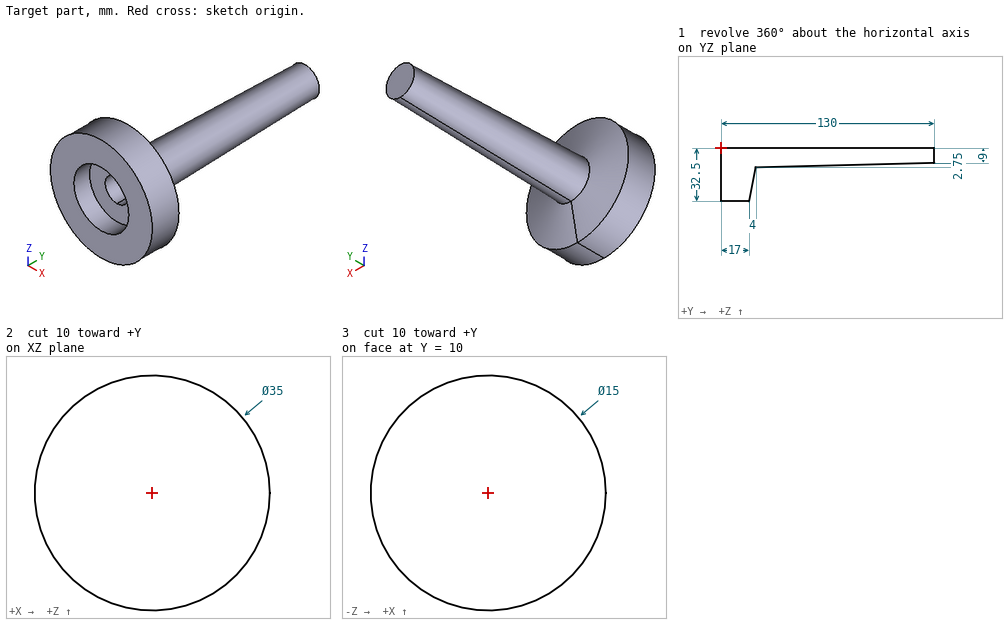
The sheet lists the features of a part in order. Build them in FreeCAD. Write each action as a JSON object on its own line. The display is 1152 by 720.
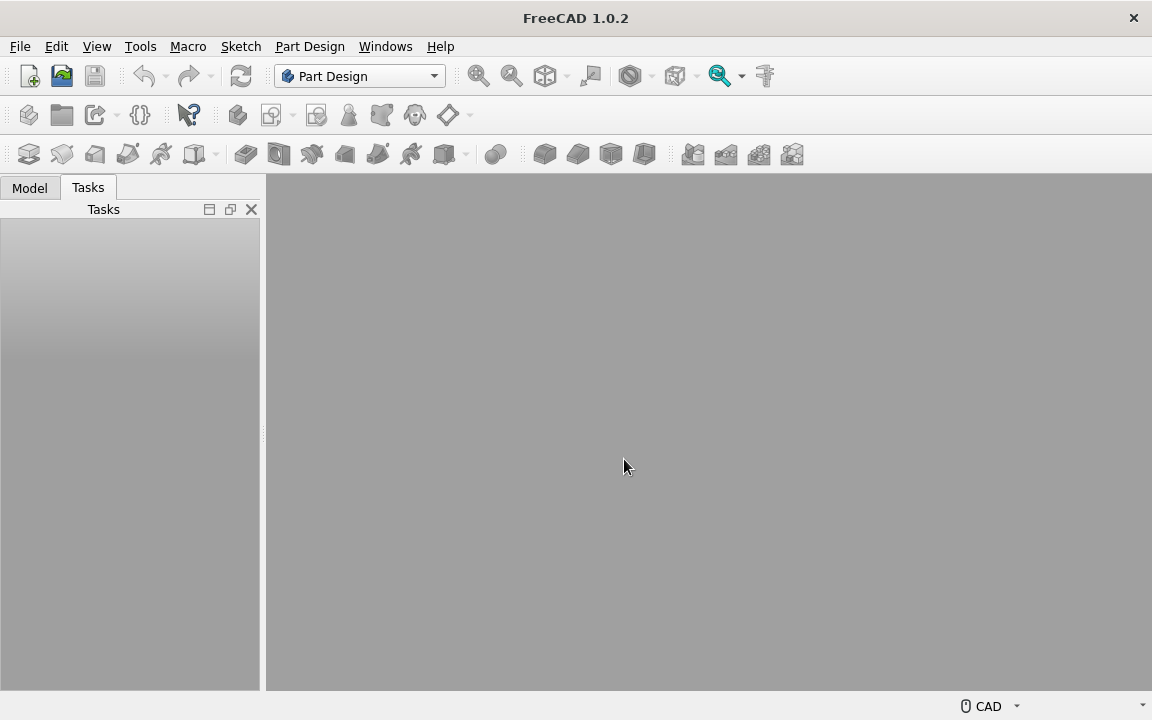
{"action": "left_click", "coordinate": [29, 76]}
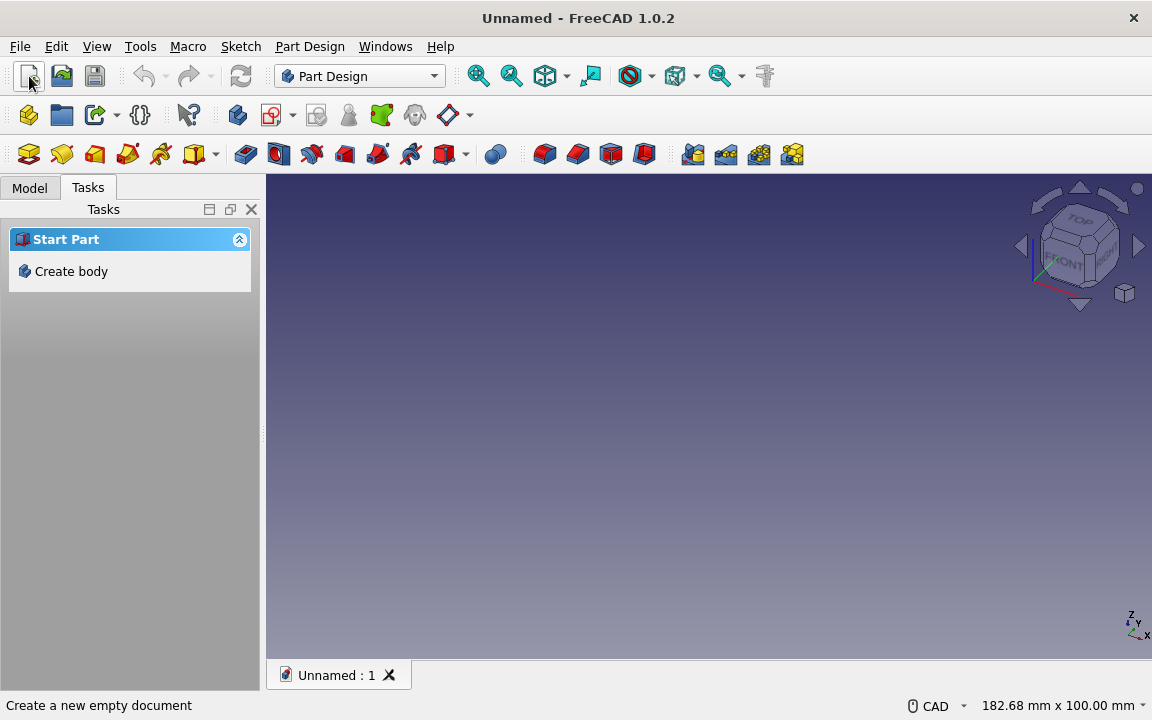
{"action": "left_click", "coordinate": [270, 116]}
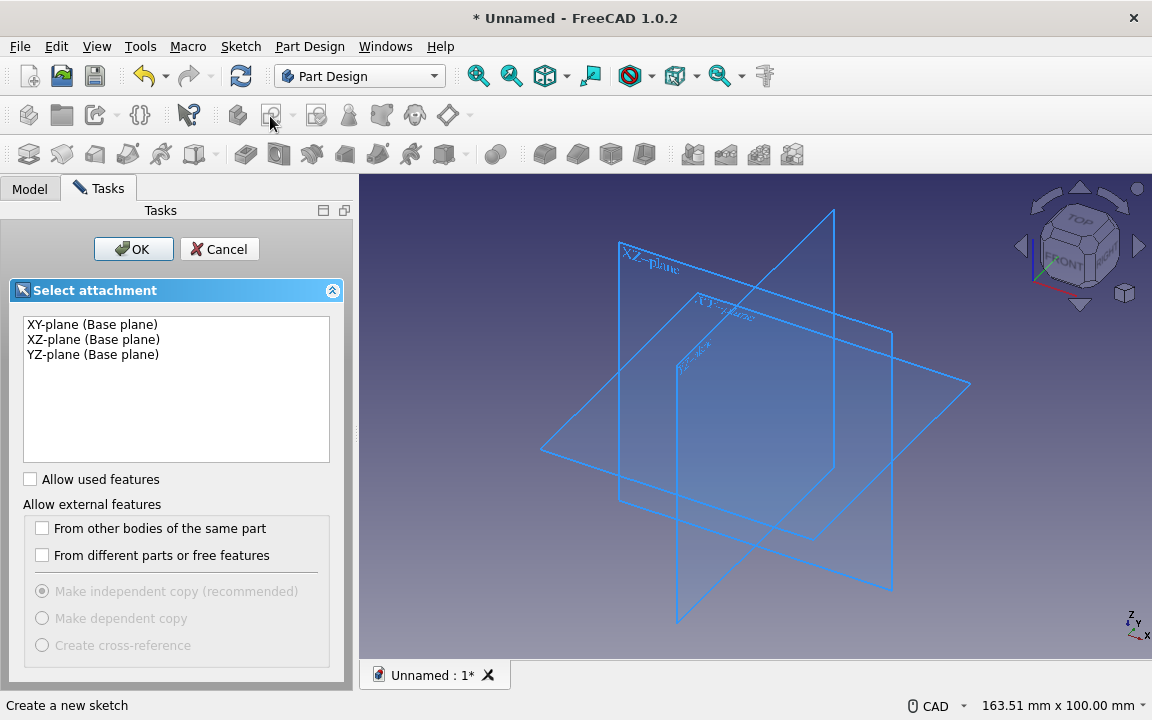
{"action": "left_click", "coordinate": [84, 354]}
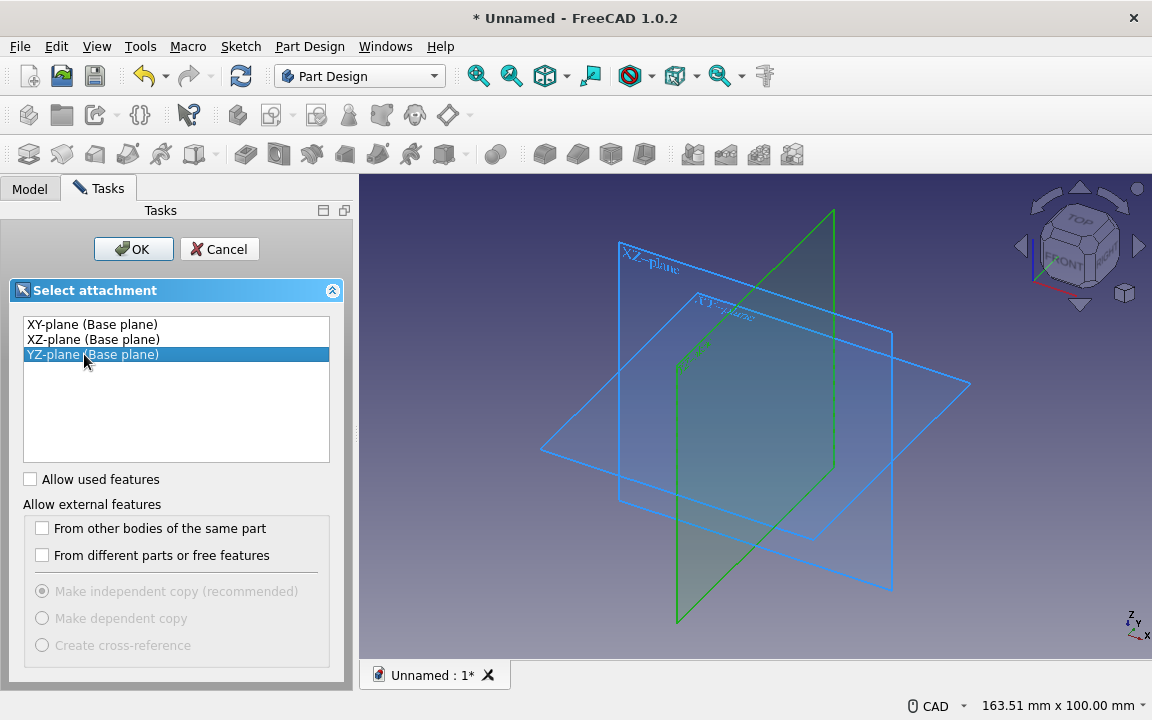
{"action": "left_click", "coordinate": [134, 249]}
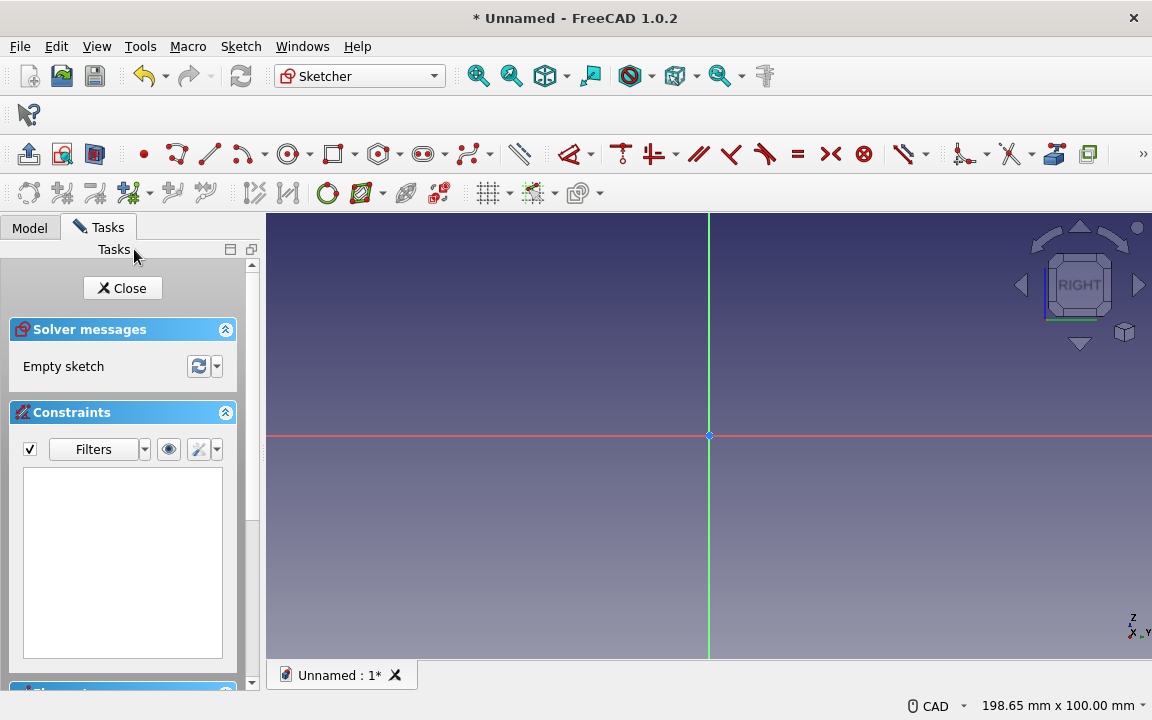
{"action": "scroll", "coordinate": [294, 289], "scroll_direction": "down", "scroll_amount": 2}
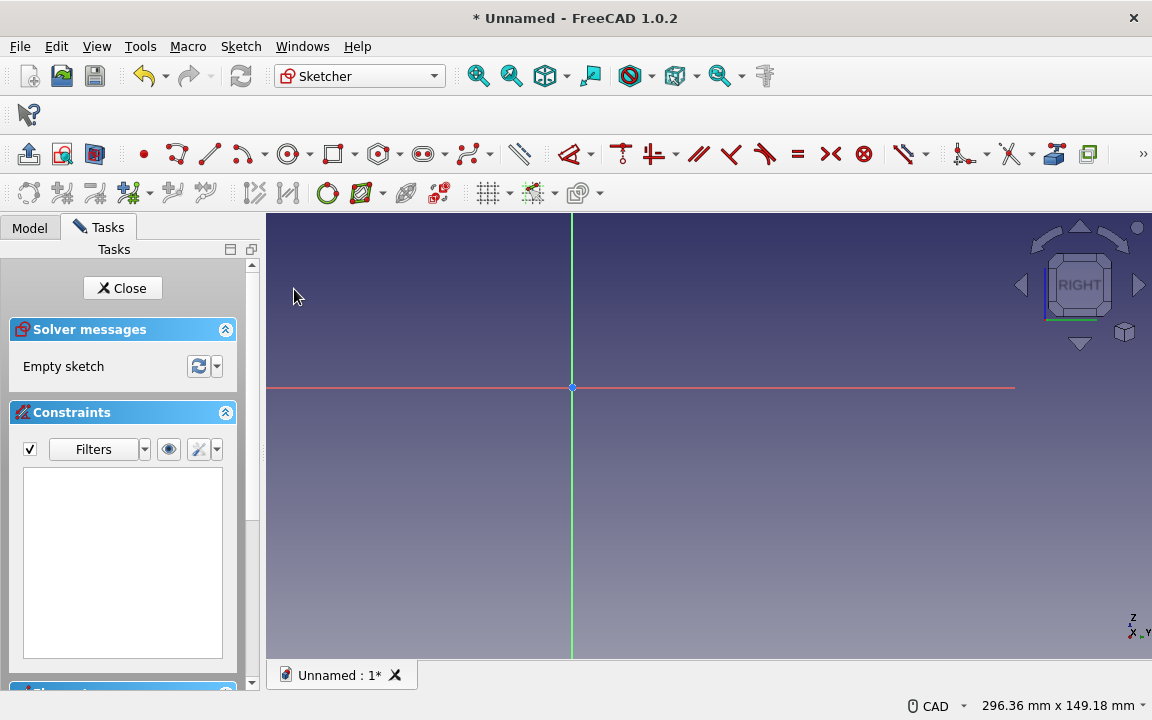
{"action": "left_click", "coordinate": [177, 154]}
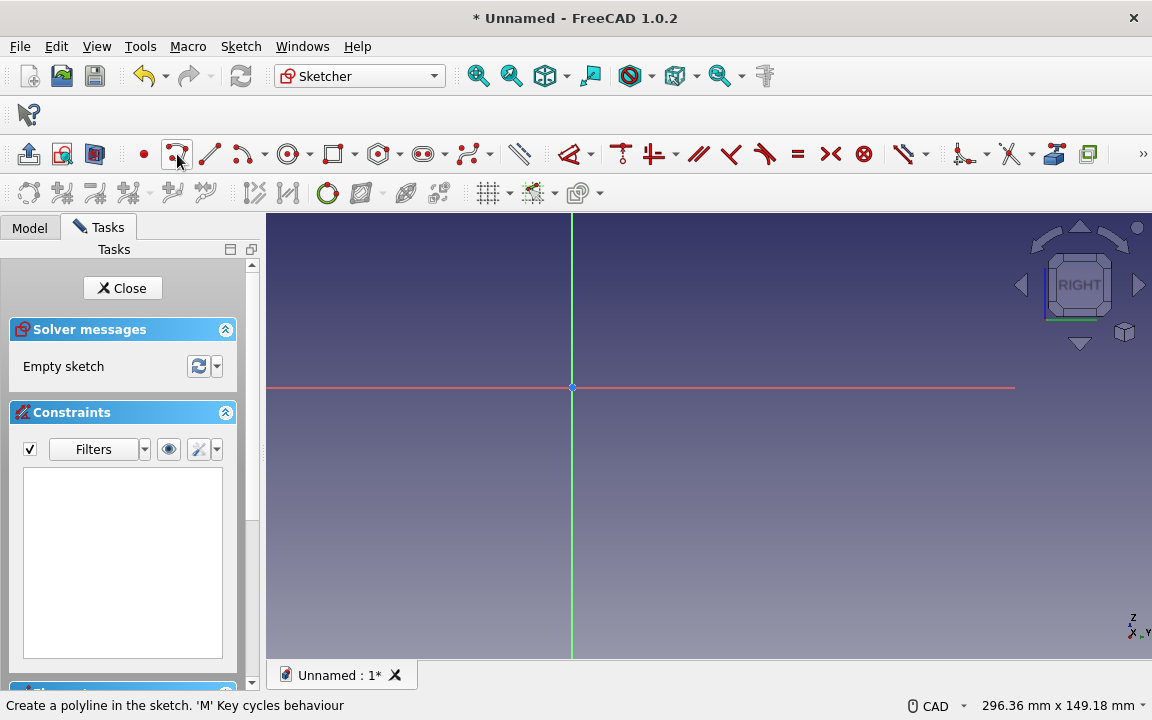
{"action": "left_click", "coordinate": [572, 388]}
{"action": "left_click", "coordinate": [581, 485]}
{"action": "left_click", "coordinate": [623, 485]}
{"action": "left_click", "coordinate": [635, 423]}
{"action": "left_click", "coordinate": [961, 407]}
{"action": "left_click", "coordinate": [961, 397]}
{"action": "left_click", "coordinate": [572, 388]}
{"action": "key", "text": "Escape"}
{"action": "key", "text": "Escape"}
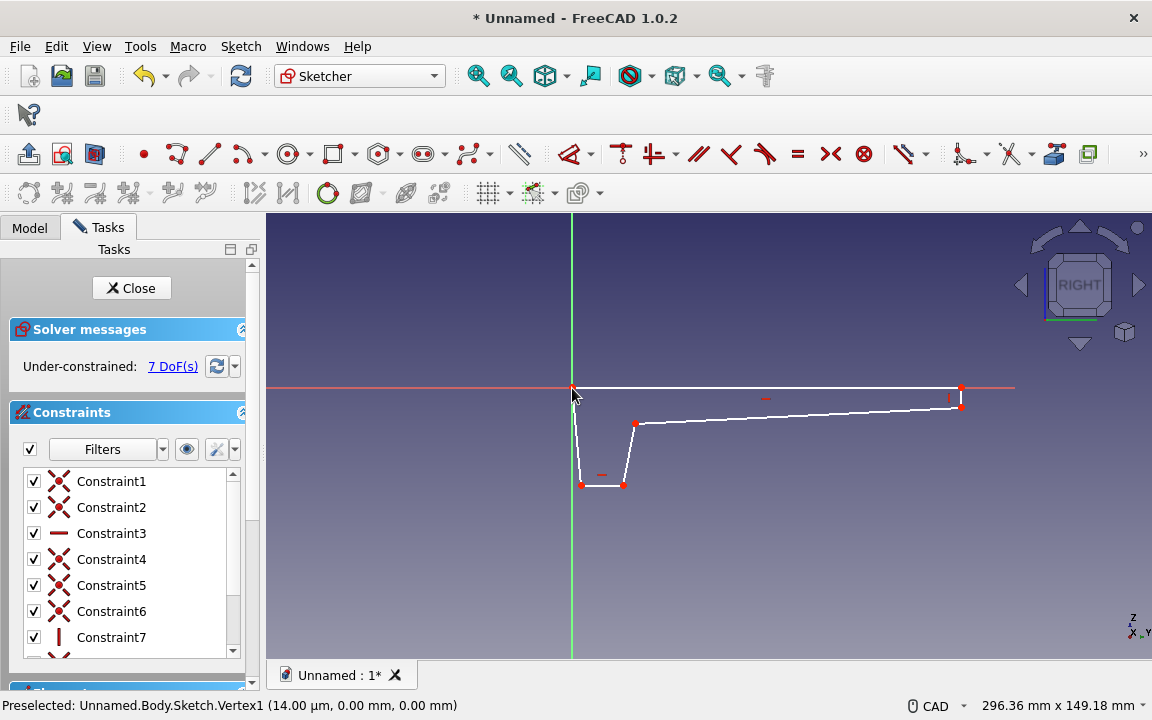
{"action": "left_click", "coordinate": [575, 417]}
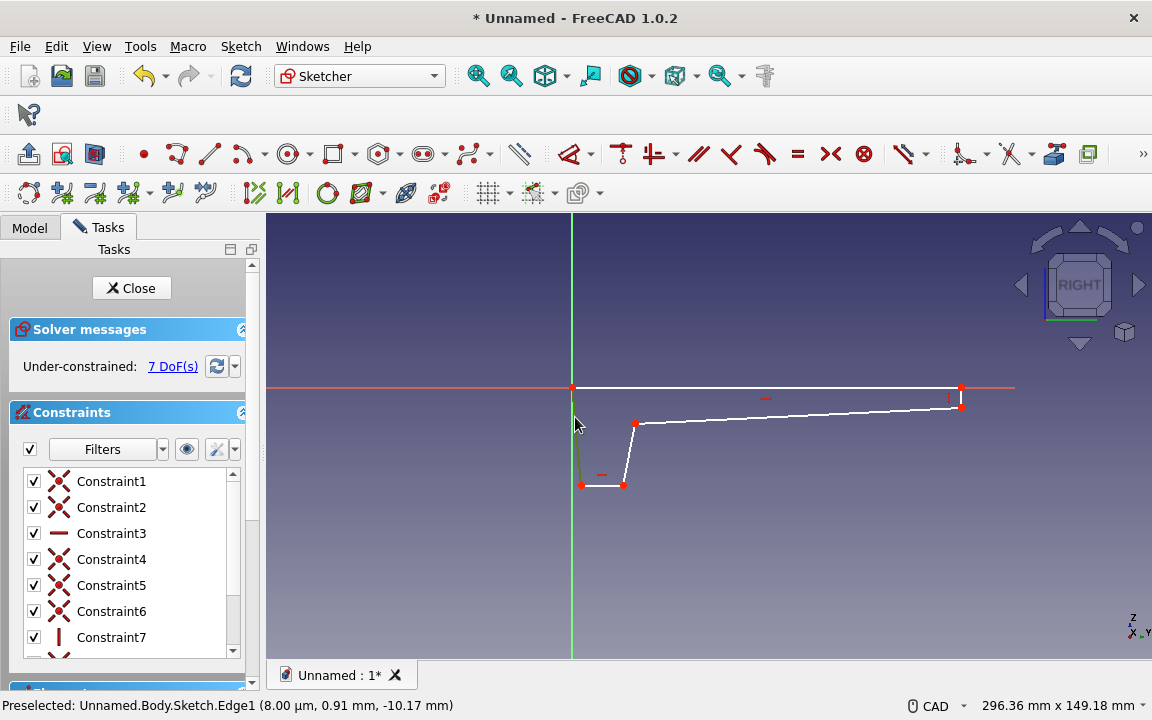
{"action": "key", "text": "v"}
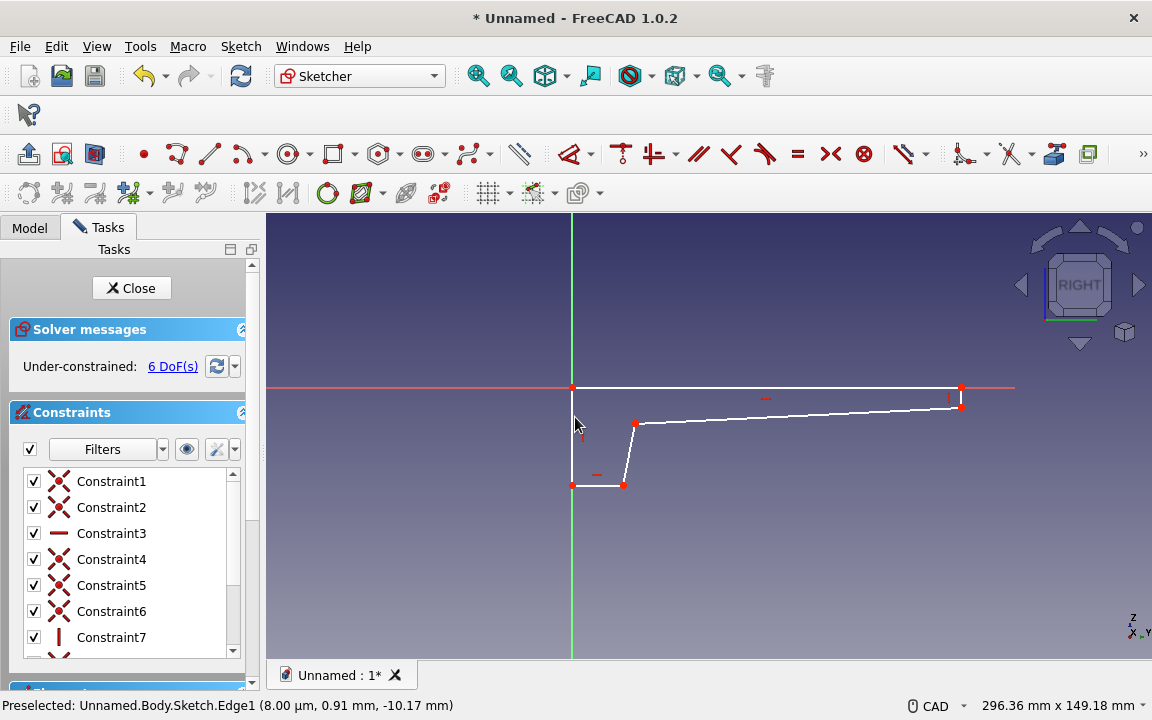
{"action": "left_click", "coordinate": [568, 154]}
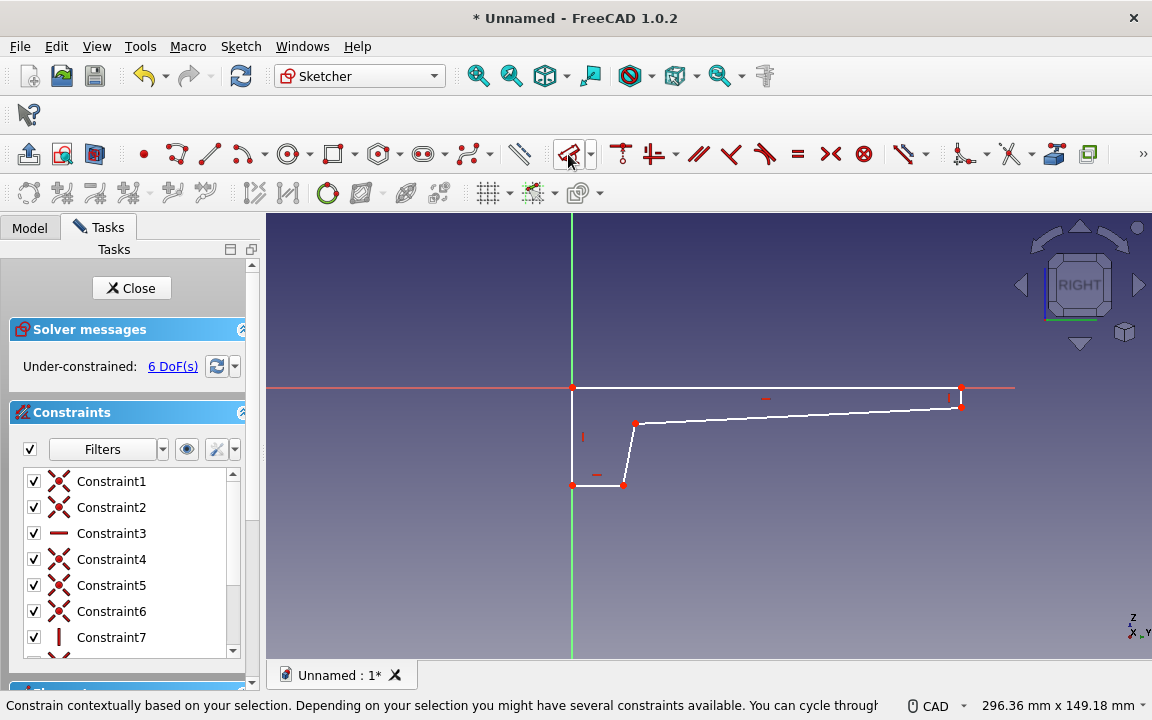
{"action": "scroll", "coordinate": [961, 398], "scroll_direction": "up", "scroll_amount": 2}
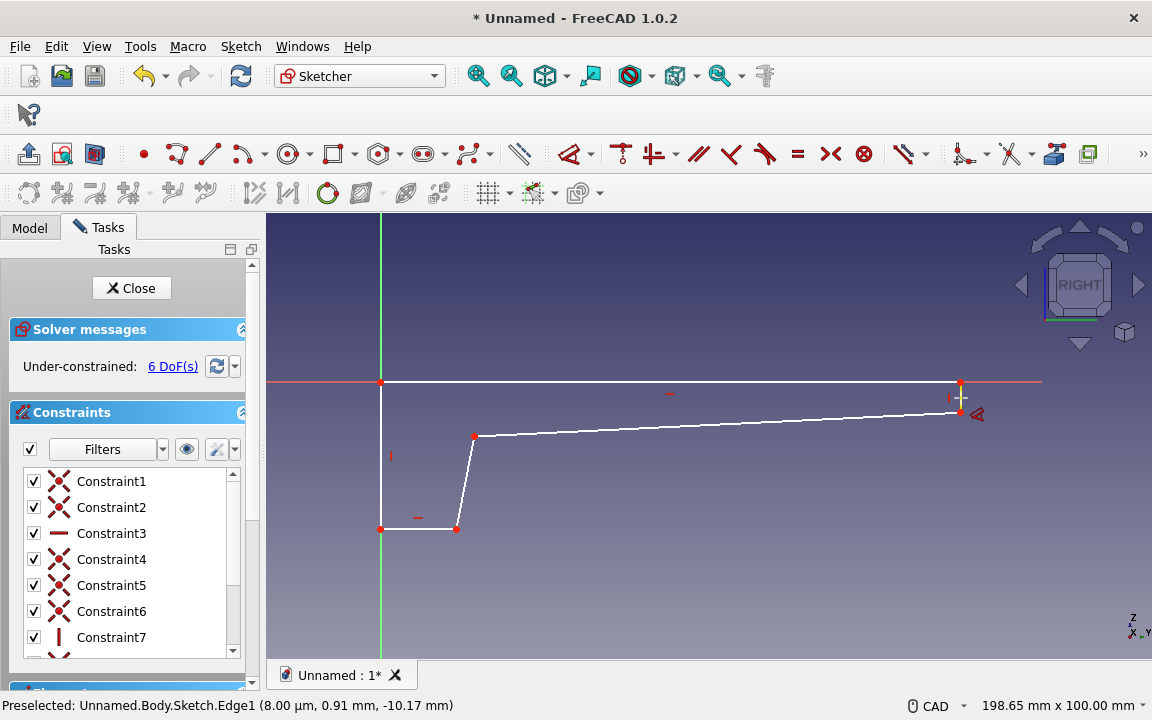
{"action": "left_click", "coordinate": [961, 397]}
{"action": "left_click", "coordinate": [927, 397]}